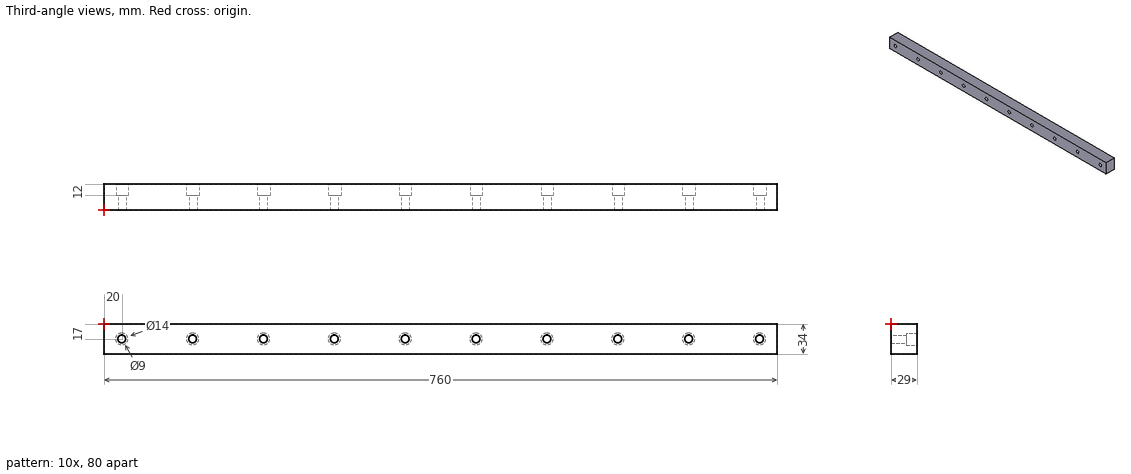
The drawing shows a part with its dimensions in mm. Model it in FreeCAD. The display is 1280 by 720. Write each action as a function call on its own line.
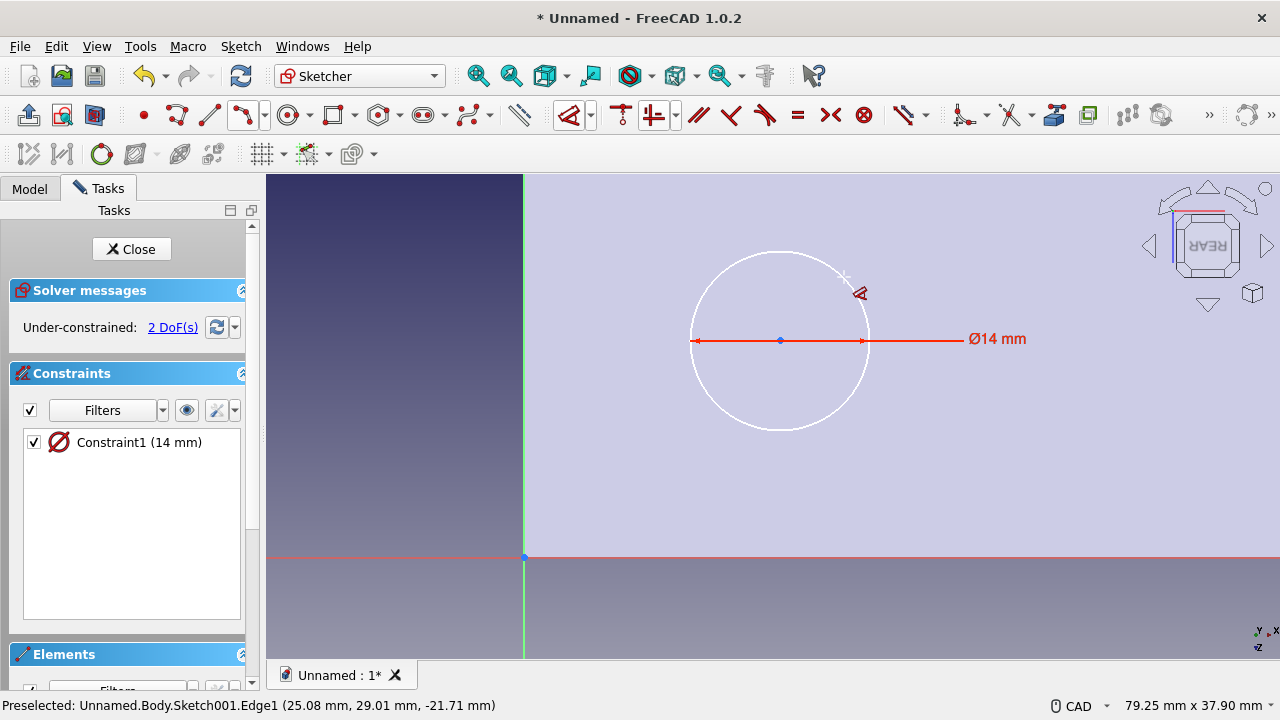
click(780, 341)
click(652, 592)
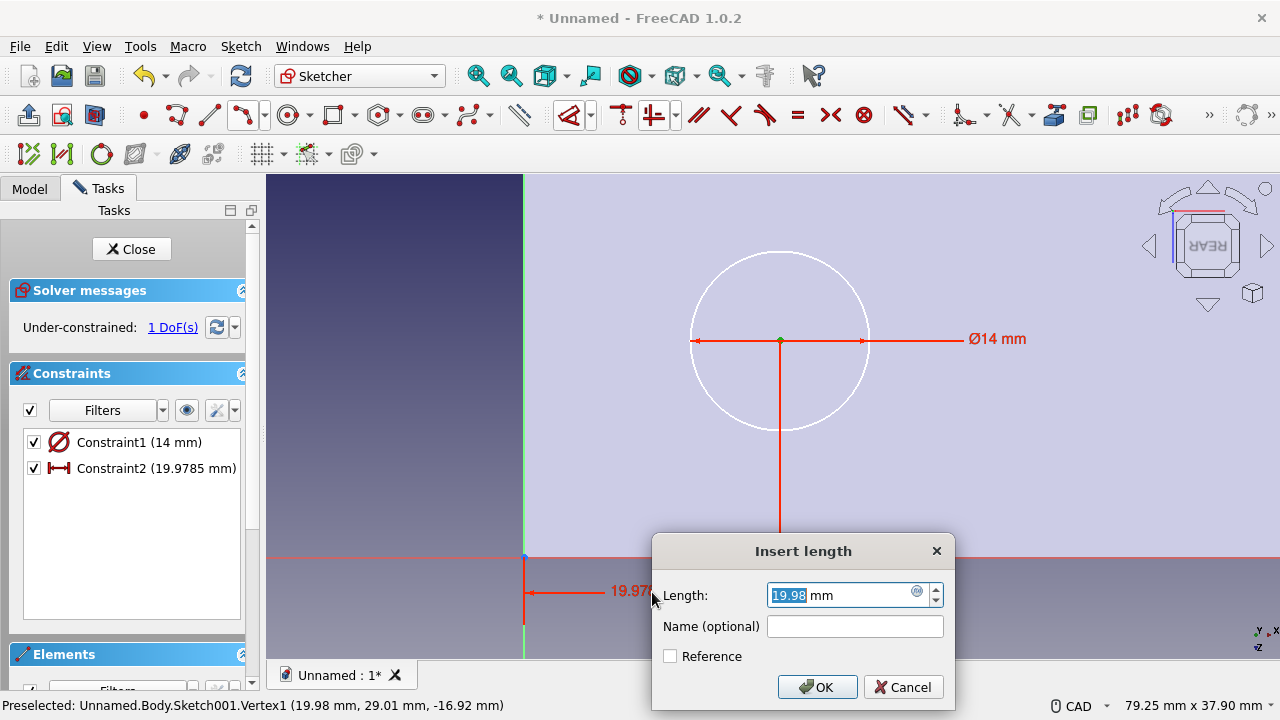
text(20)
key(Return)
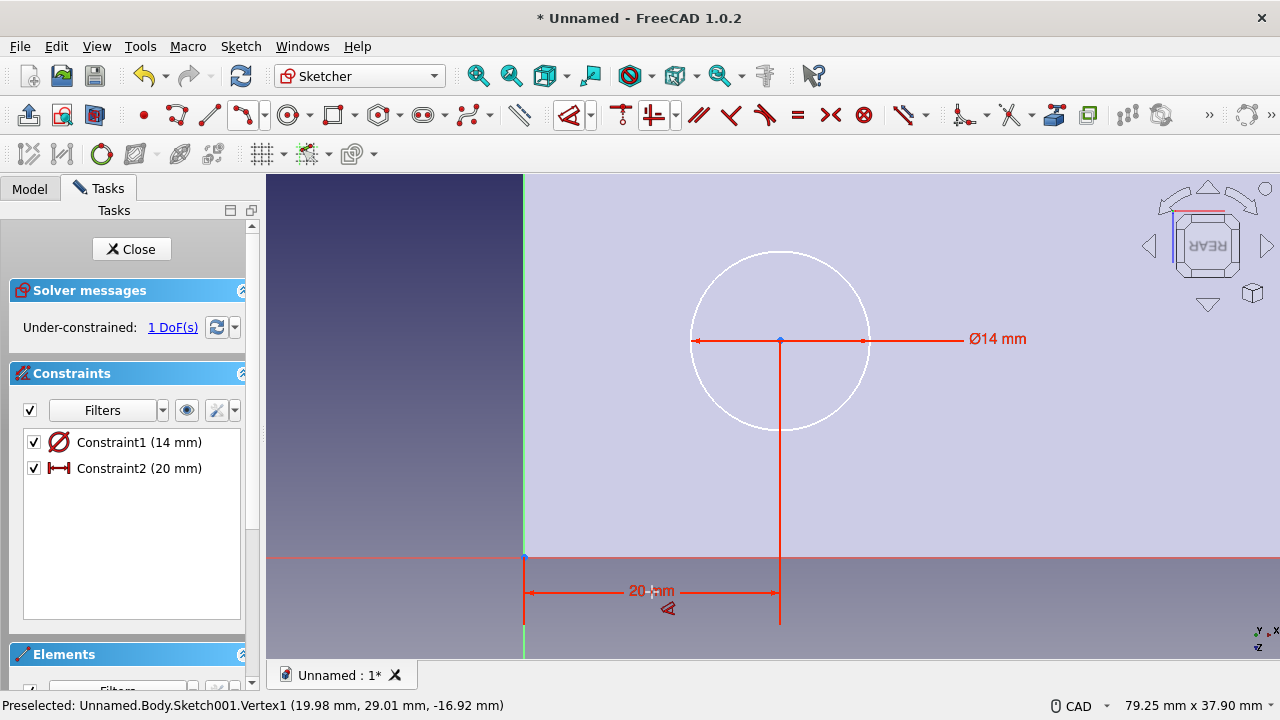
click(780, 341)
click(490, 449)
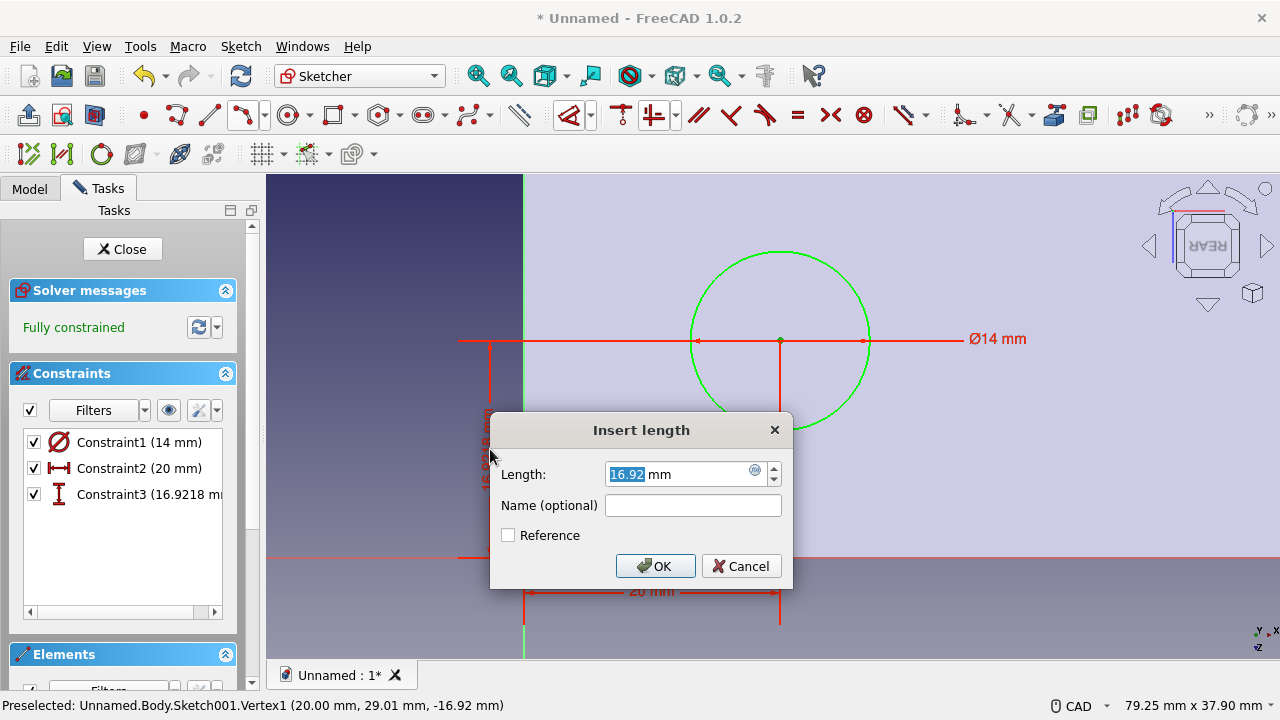
text(17)
key(Return)
key(Escape)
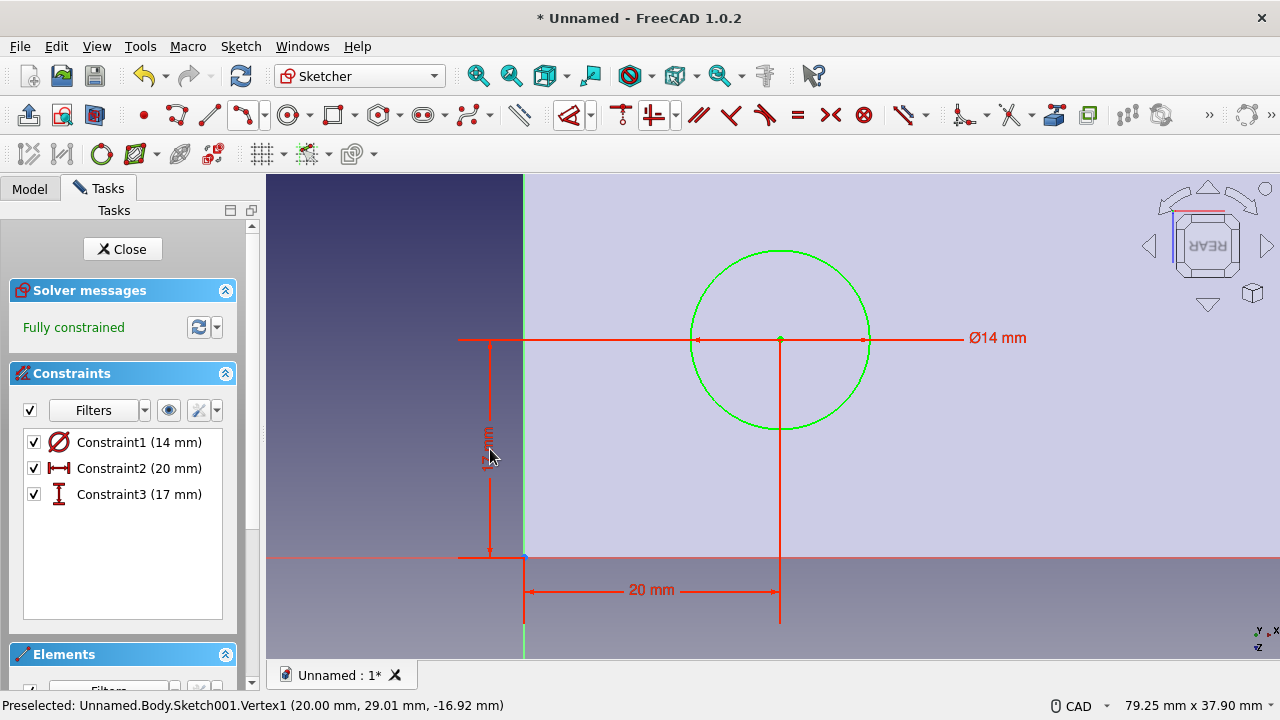
click(123, 249)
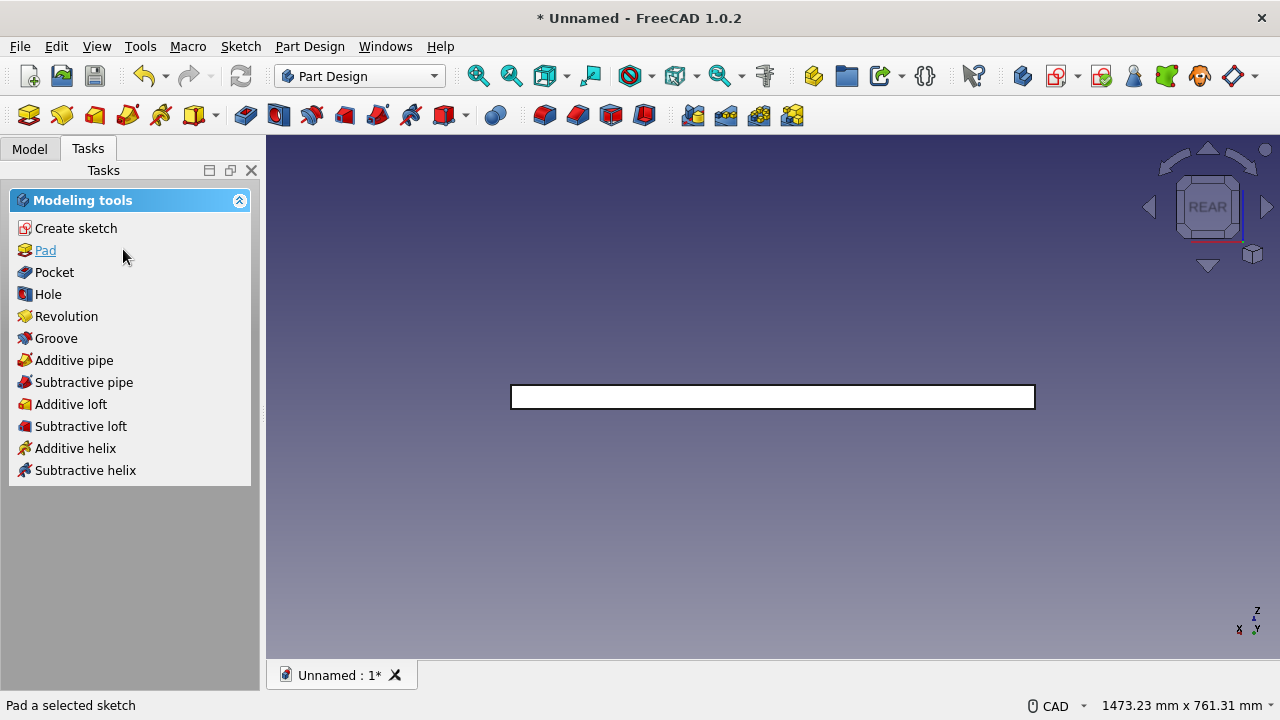
click(246, 116)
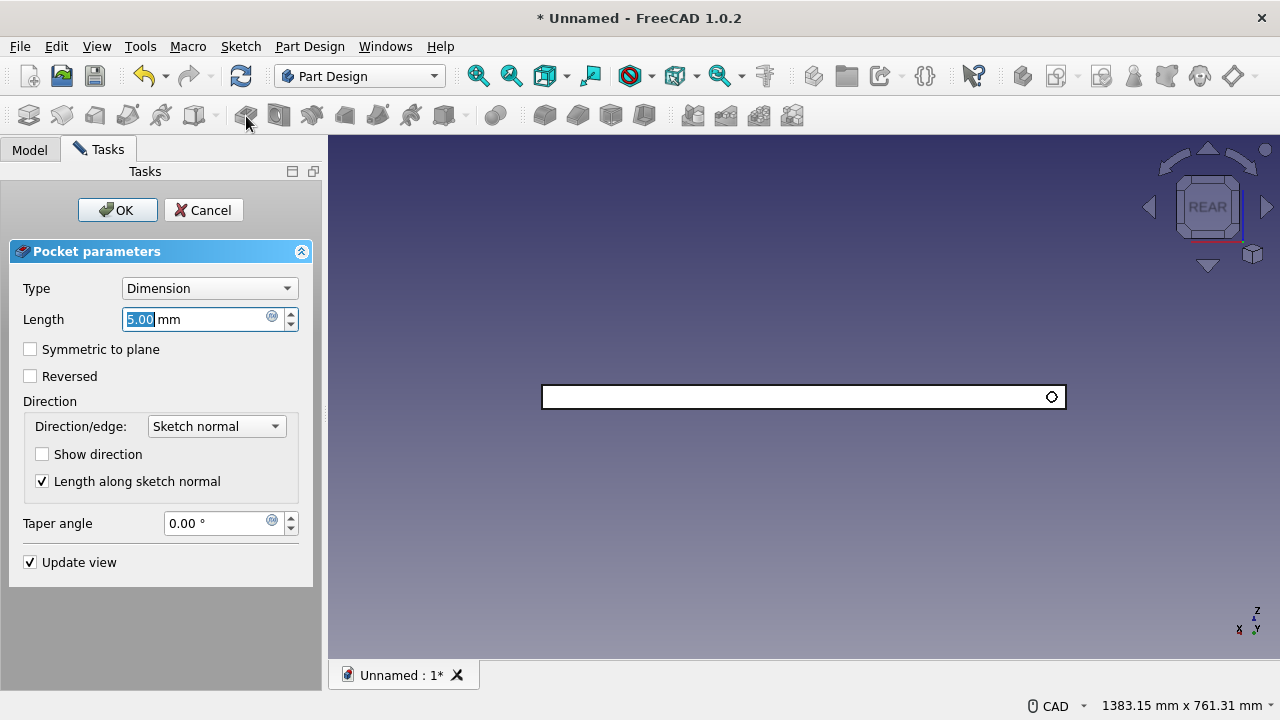
text(12)
key(Tab)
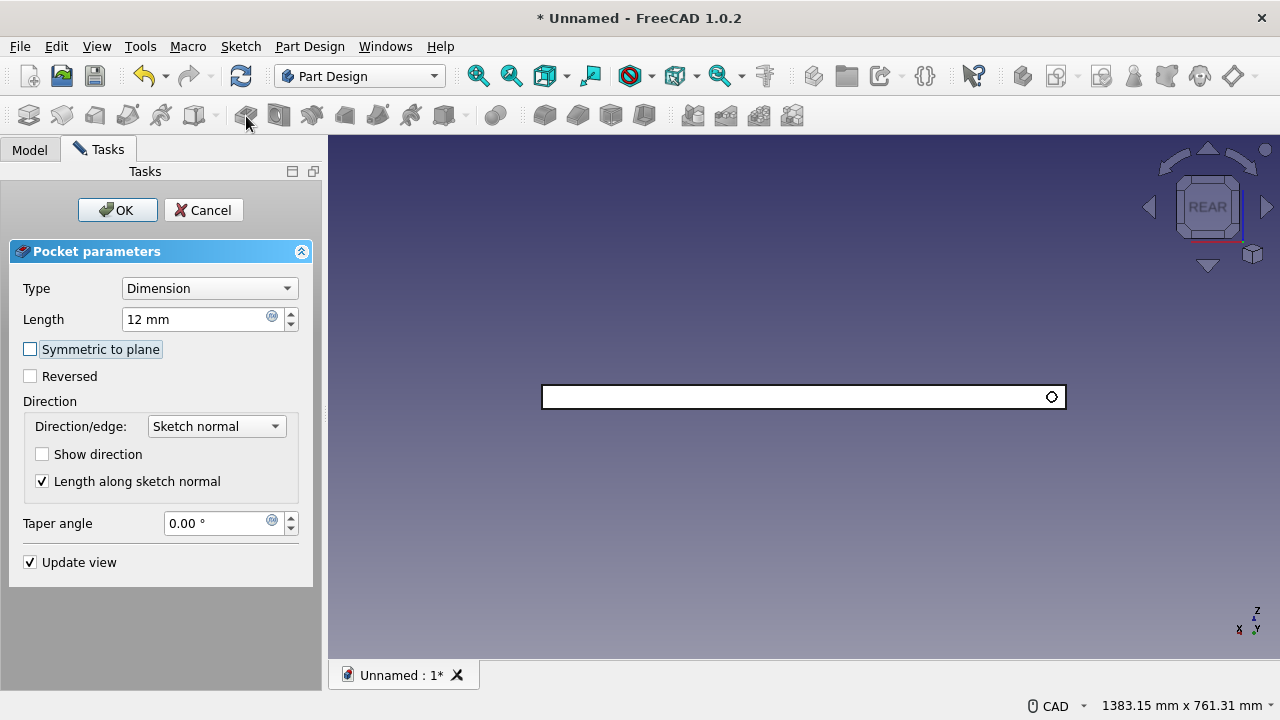
click(118, 210)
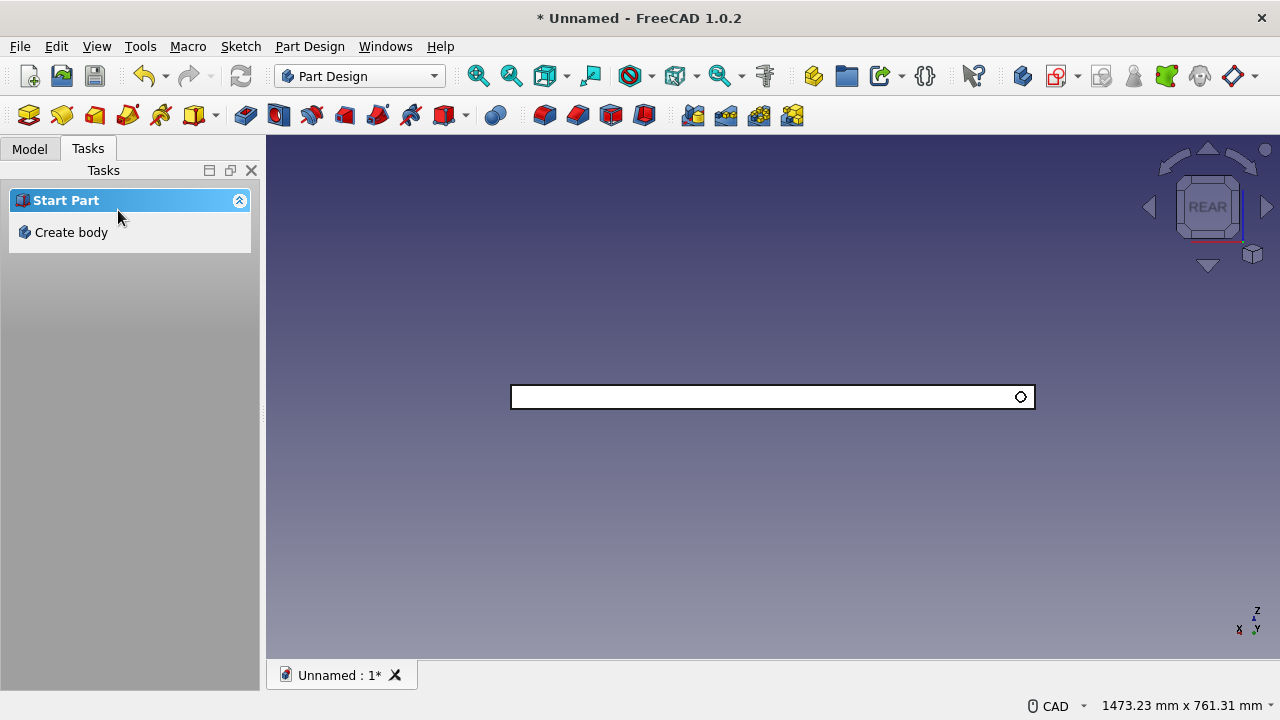
scroll(1021, 396, up, 5)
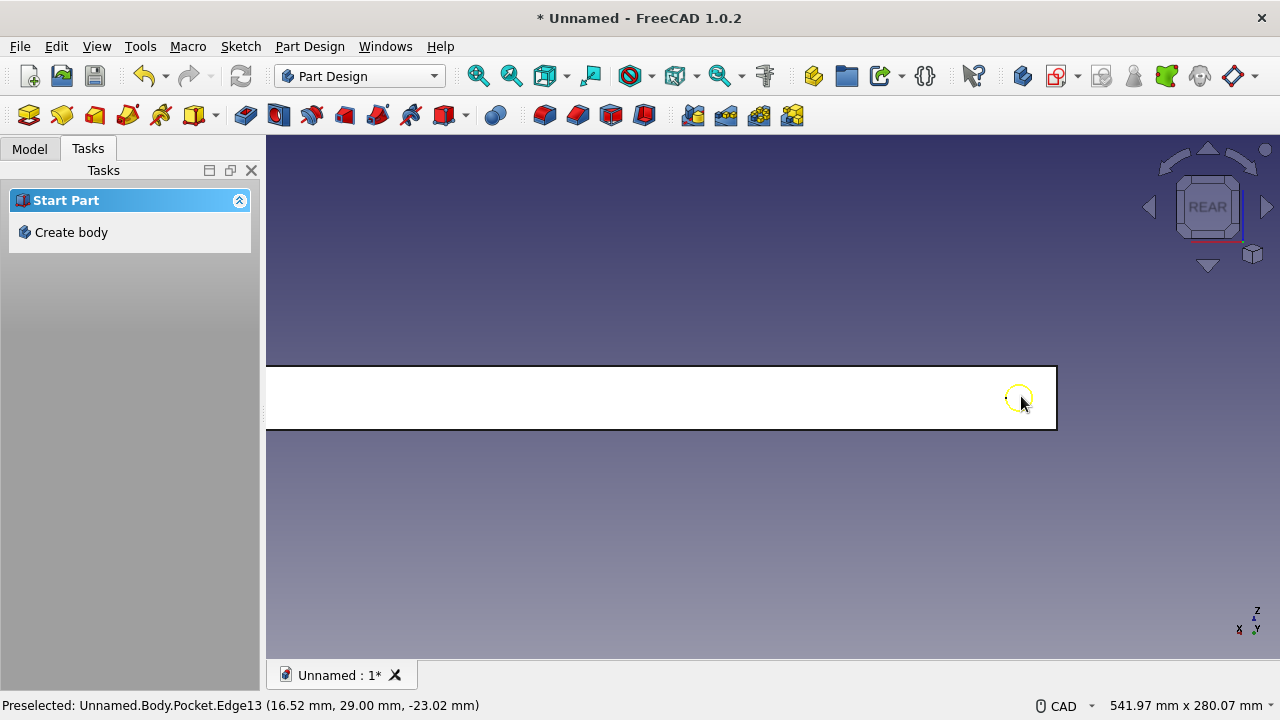
click(1019, 397)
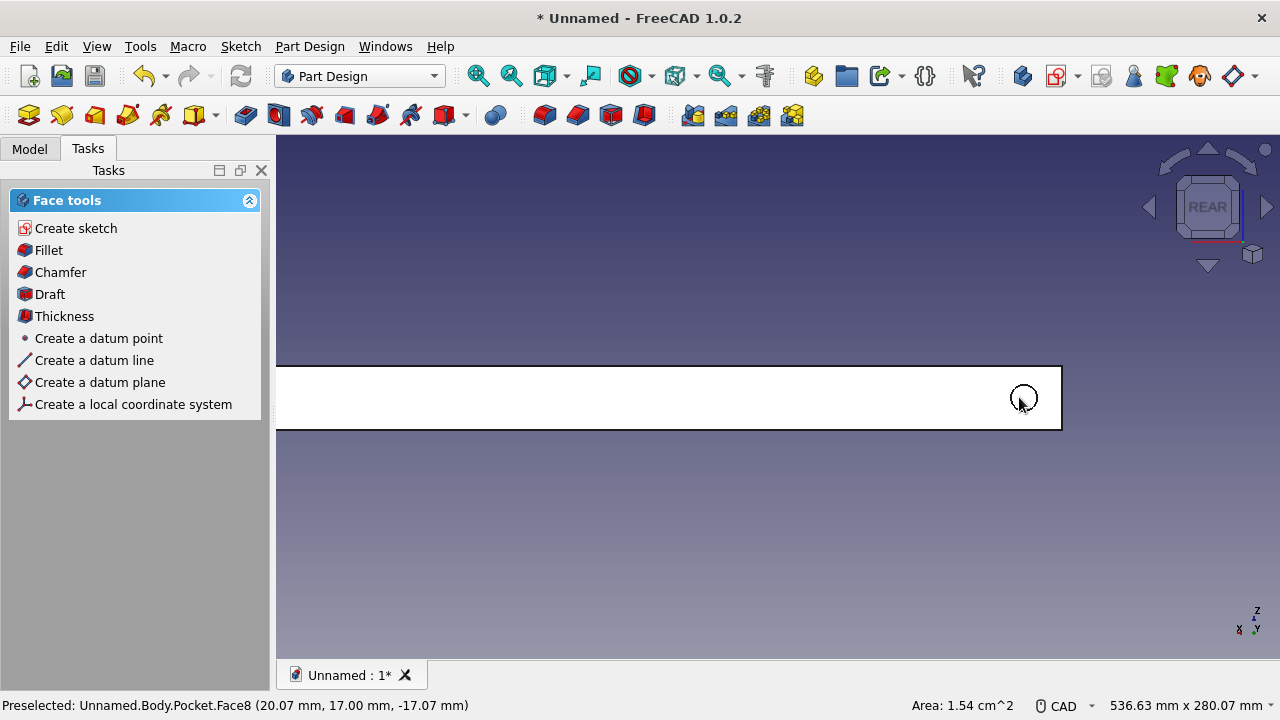
click(1056, 76)